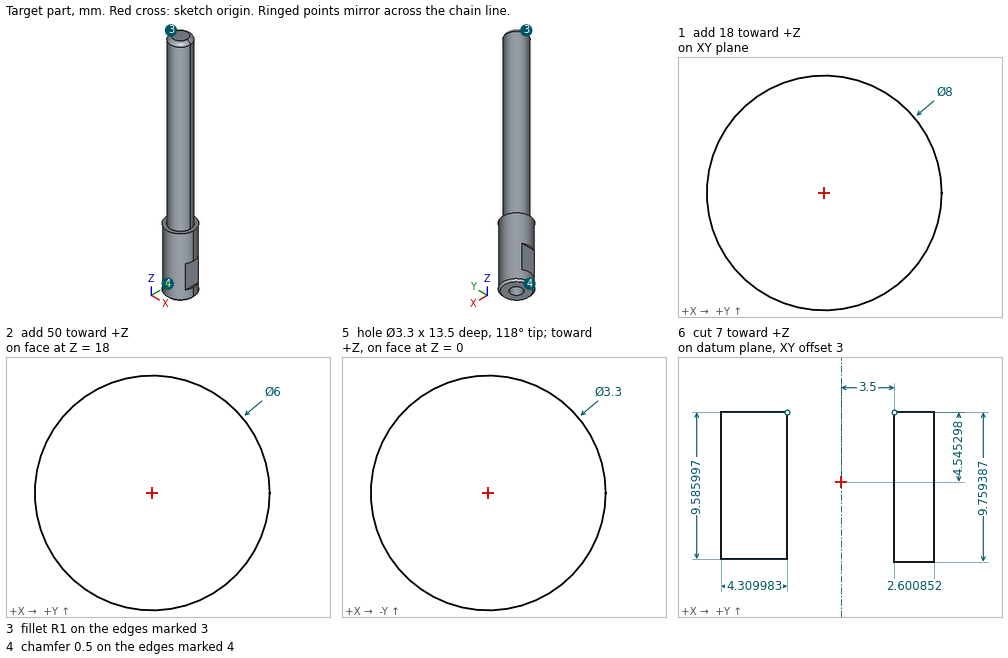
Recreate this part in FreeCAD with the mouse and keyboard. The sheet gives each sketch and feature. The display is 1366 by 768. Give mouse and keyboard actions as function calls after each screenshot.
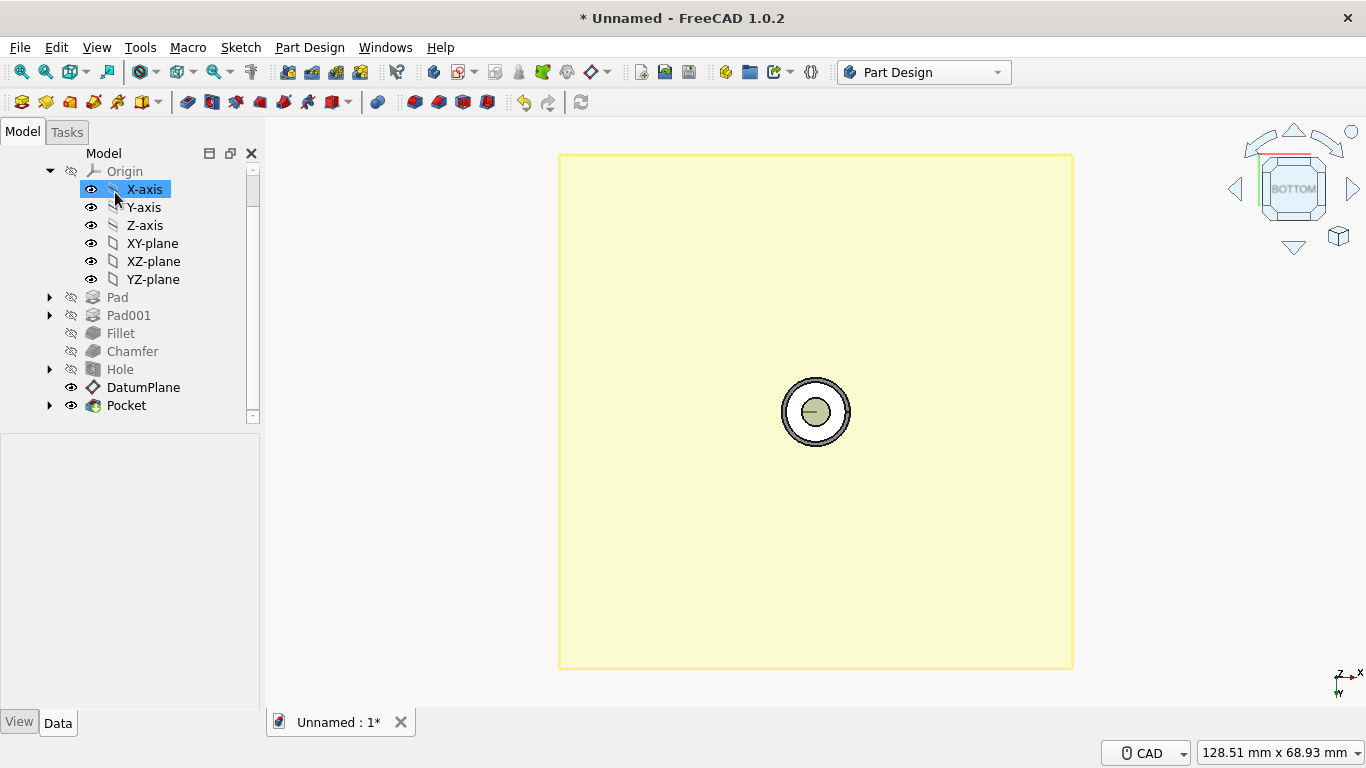
click(116, 387)
key(space)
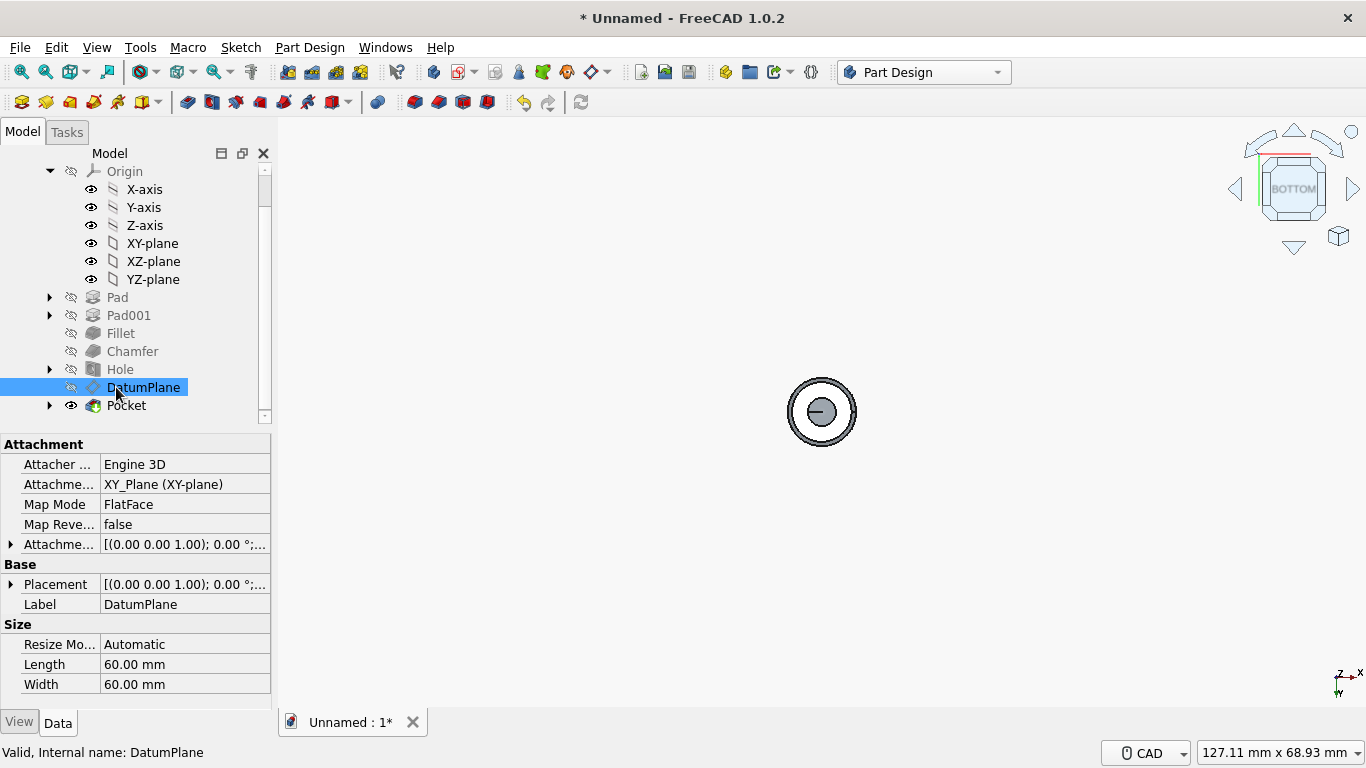
key(0)